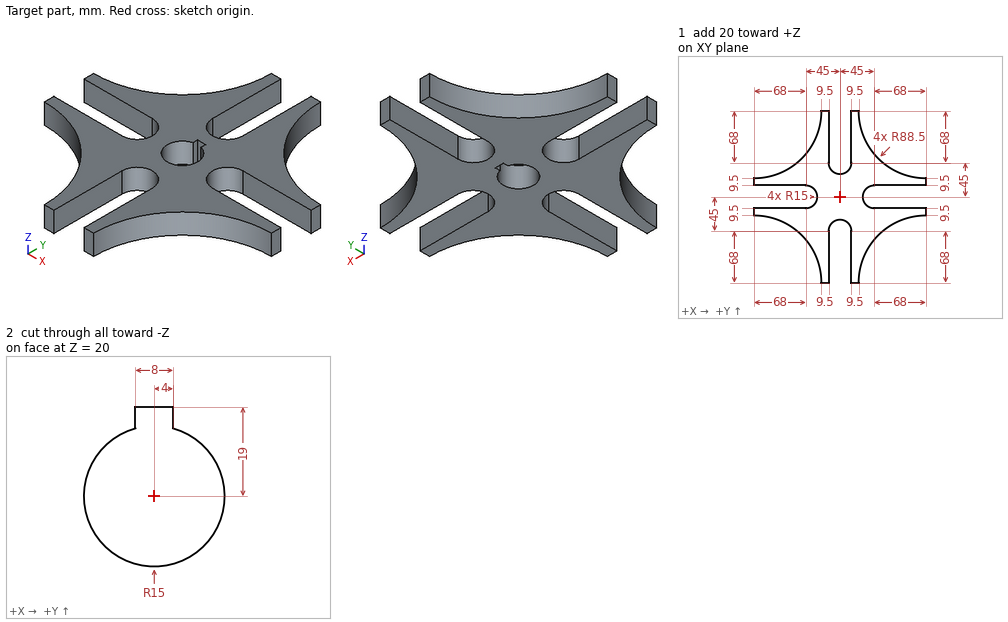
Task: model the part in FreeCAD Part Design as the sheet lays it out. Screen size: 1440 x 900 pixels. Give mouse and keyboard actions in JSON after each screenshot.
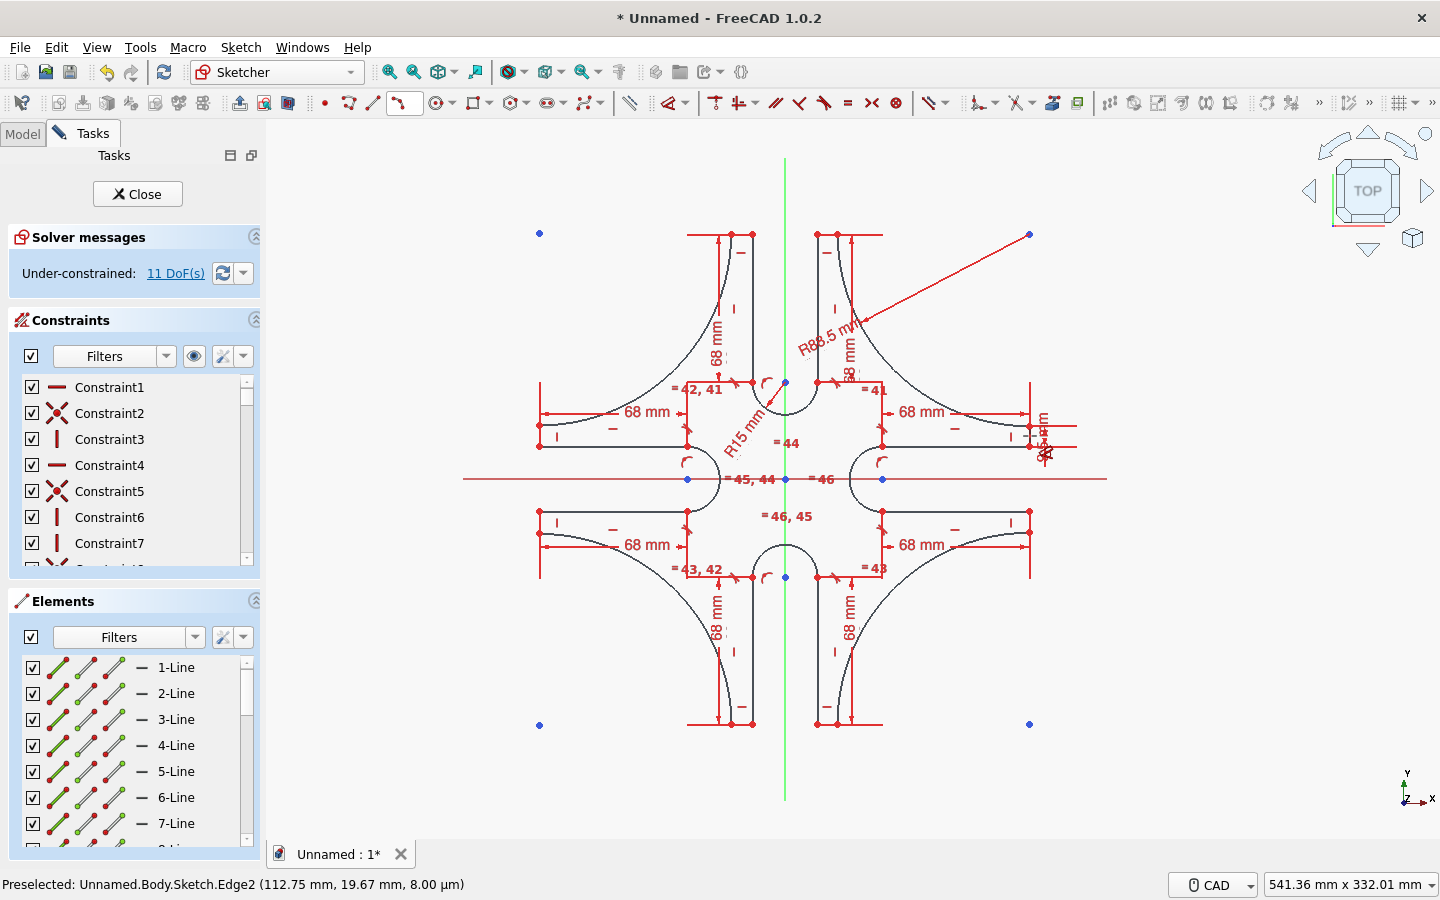
{"action": "scroll", "coordinate": [832, 235], "scroll_direction": "up", "scroll_amount": 5}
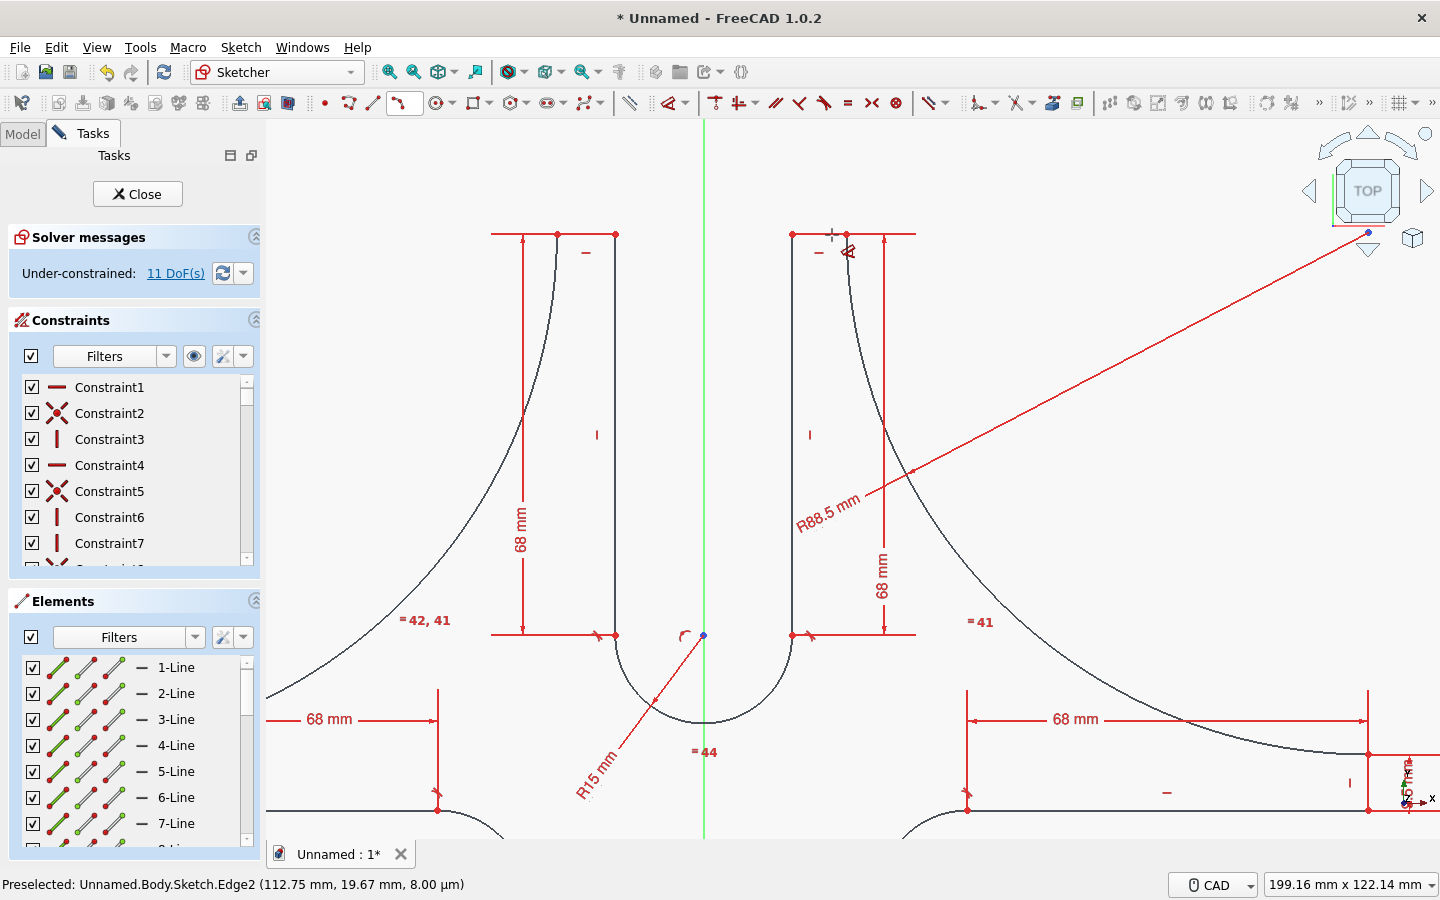
{"action": "left_click", "coordinate": [830, 234]}
{"action": "left_click", "coordinate": [819, 200]}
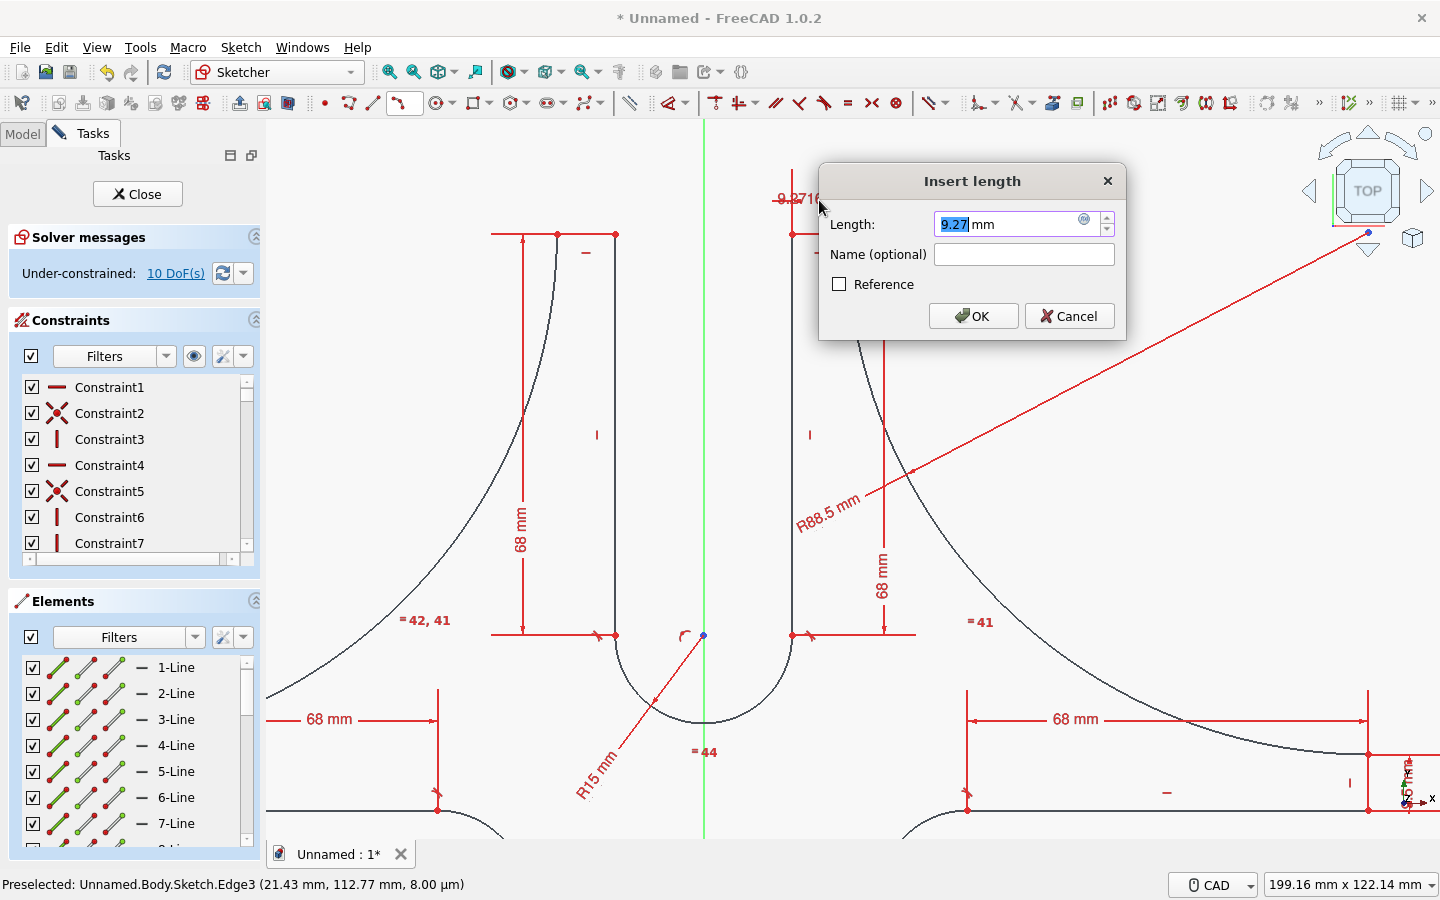
{"action": "type", "text": "9.5"}
{"action": "key", "text": "Return"}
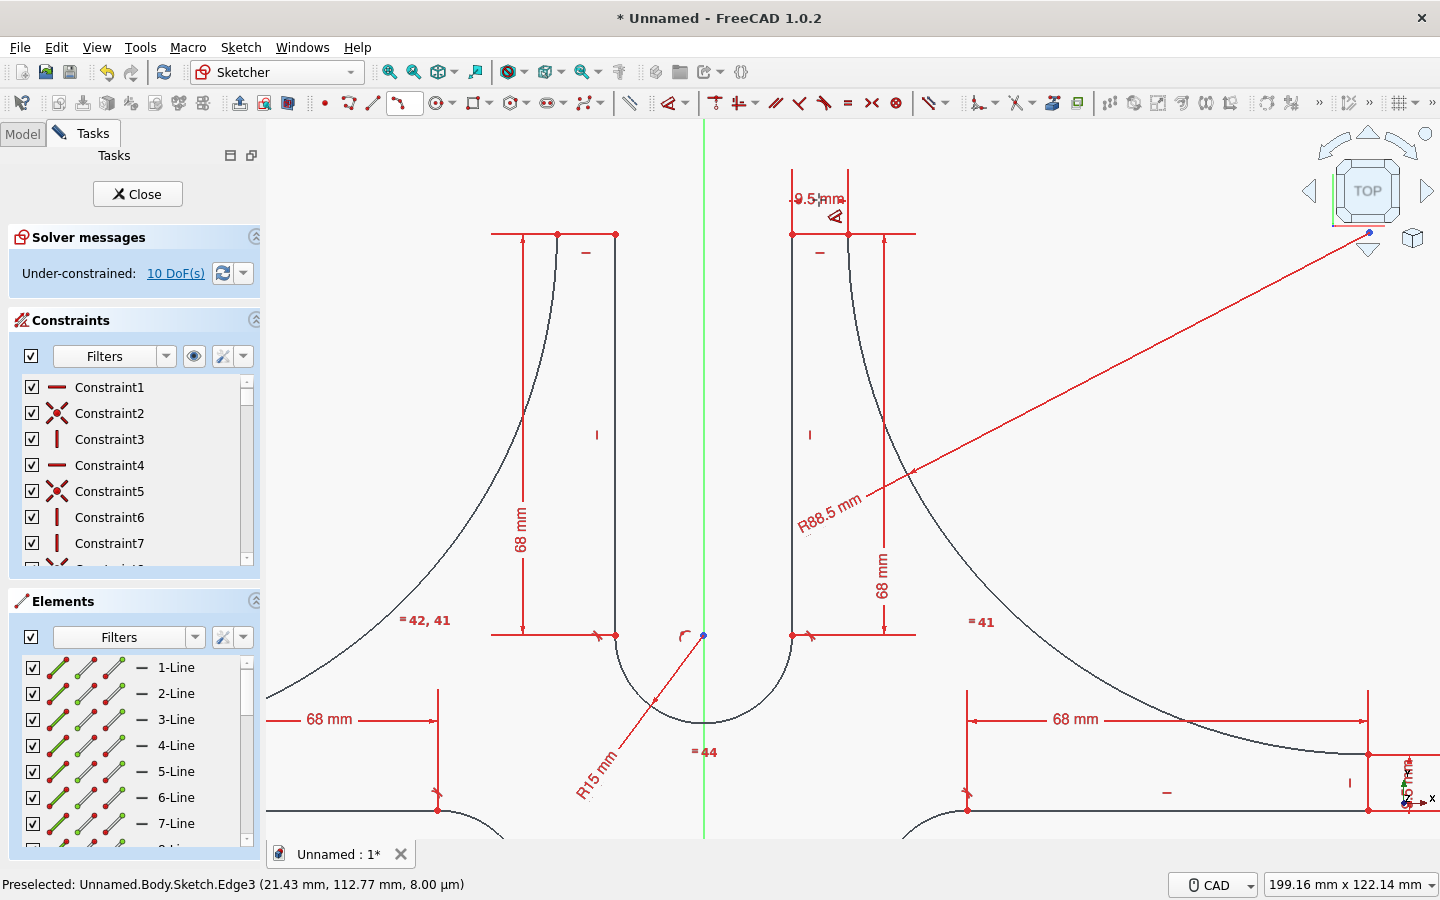
{"action": "left_click", "coordinate": [598, 234]}
{"action": "left_click", "coordinate": [586, 200]}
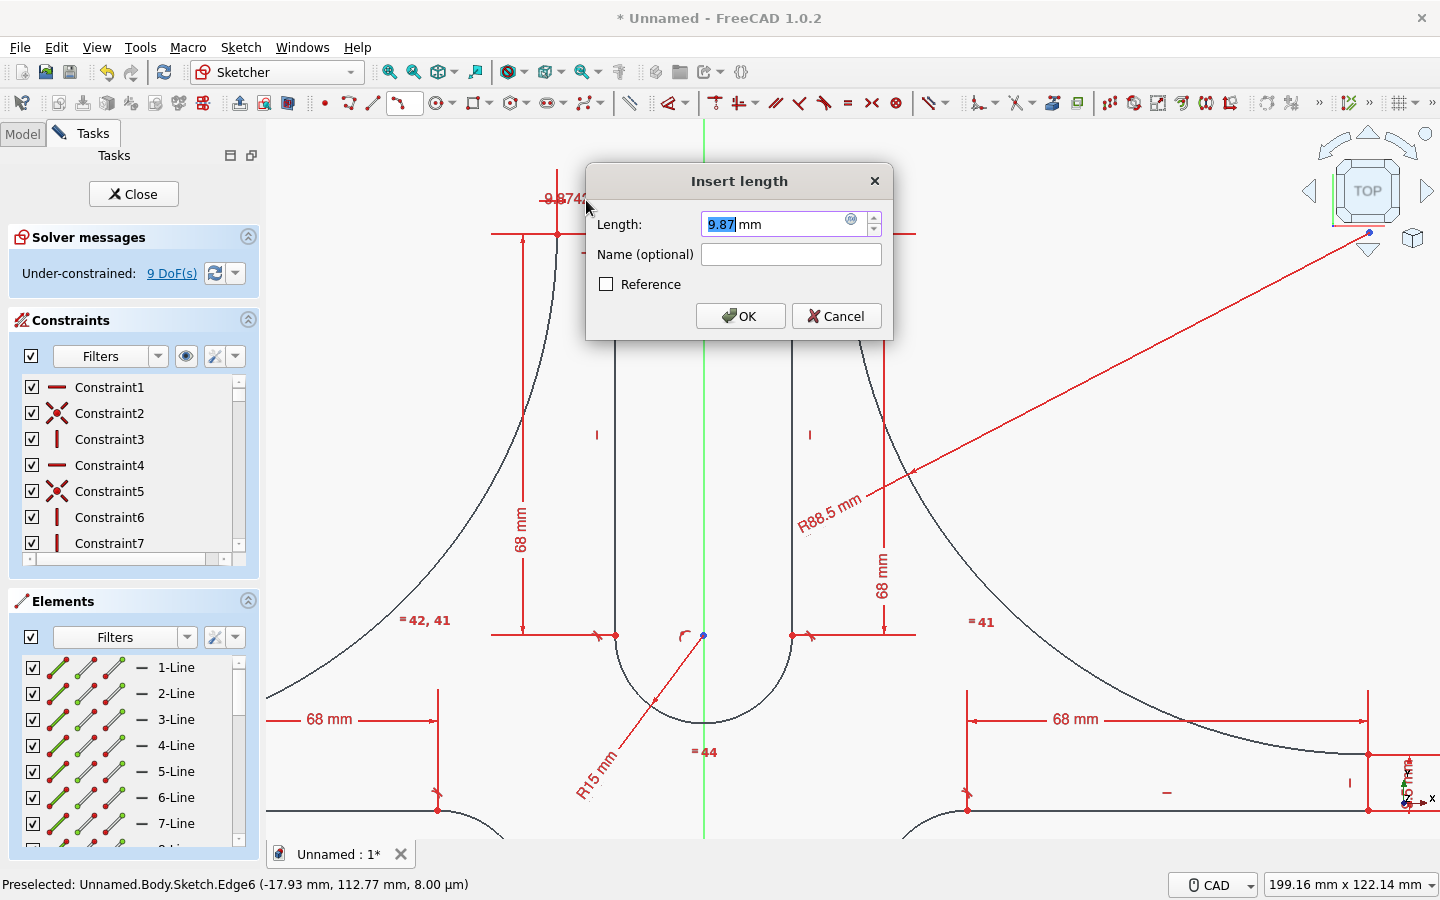
{"action": "type", "text": "9.5"}
{"action": "key", "text": "Return"}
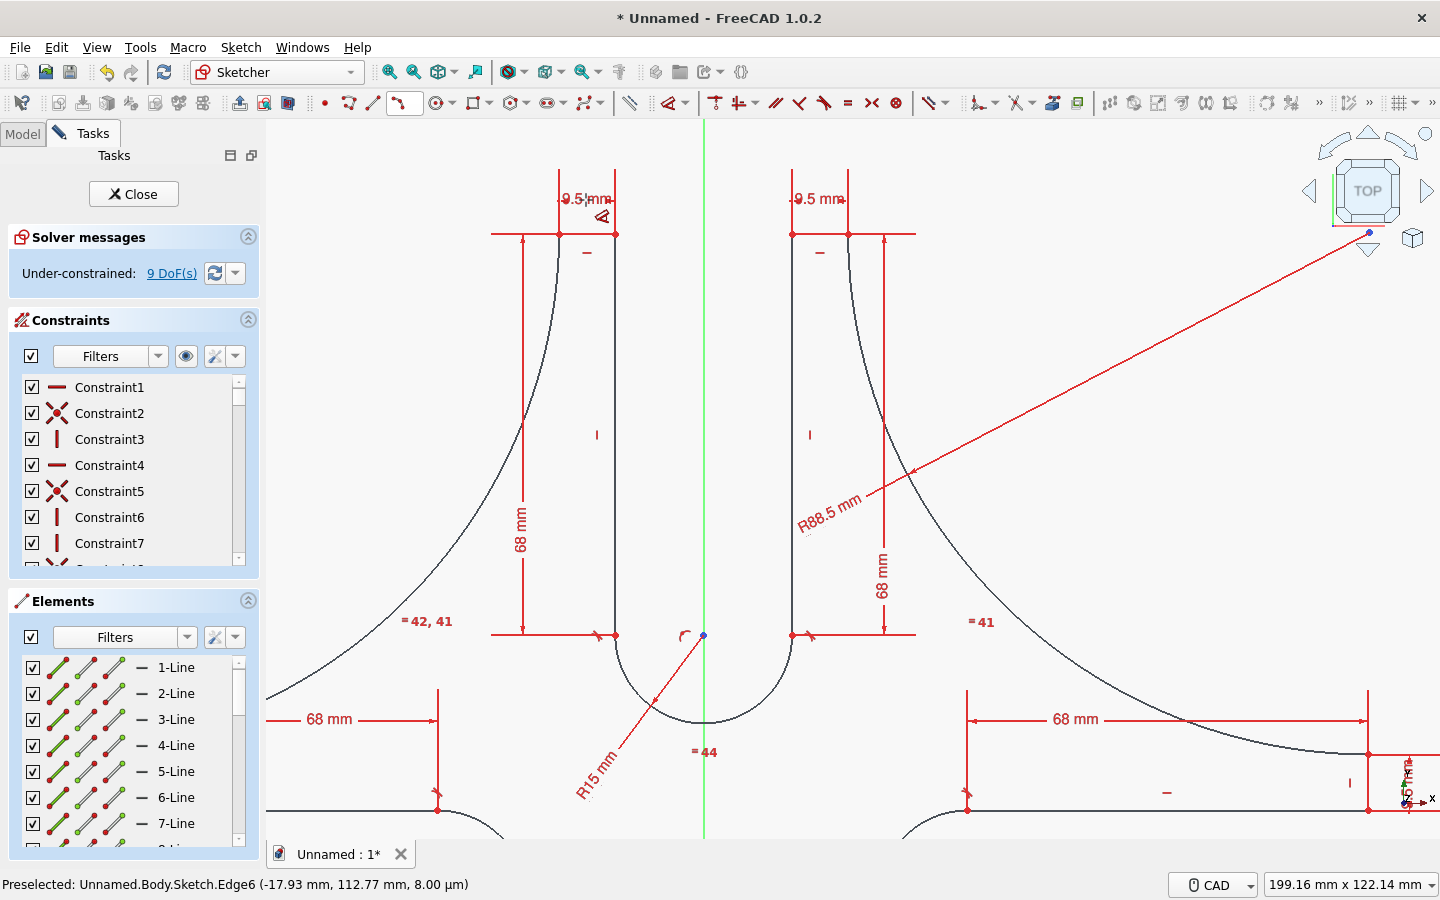
{"action": "scroll", "coordinate": [832, 235], "scroll_direction": "down", "scroll_amount": 5}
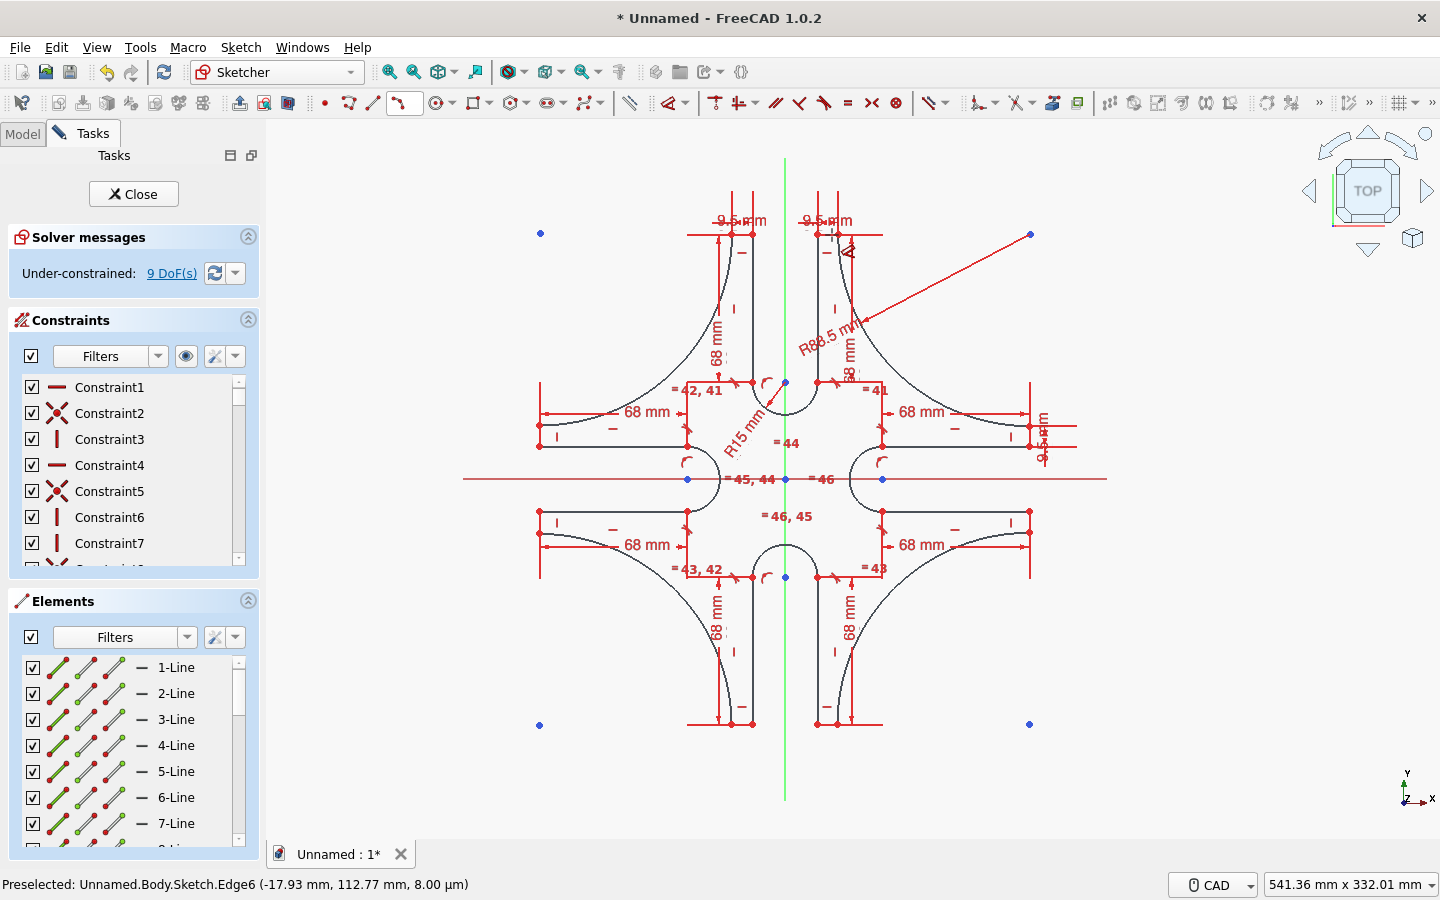
{"action": "scroll", "coordinate": [540, 432], "scroll_direction": "up", "scroll_amount": 4}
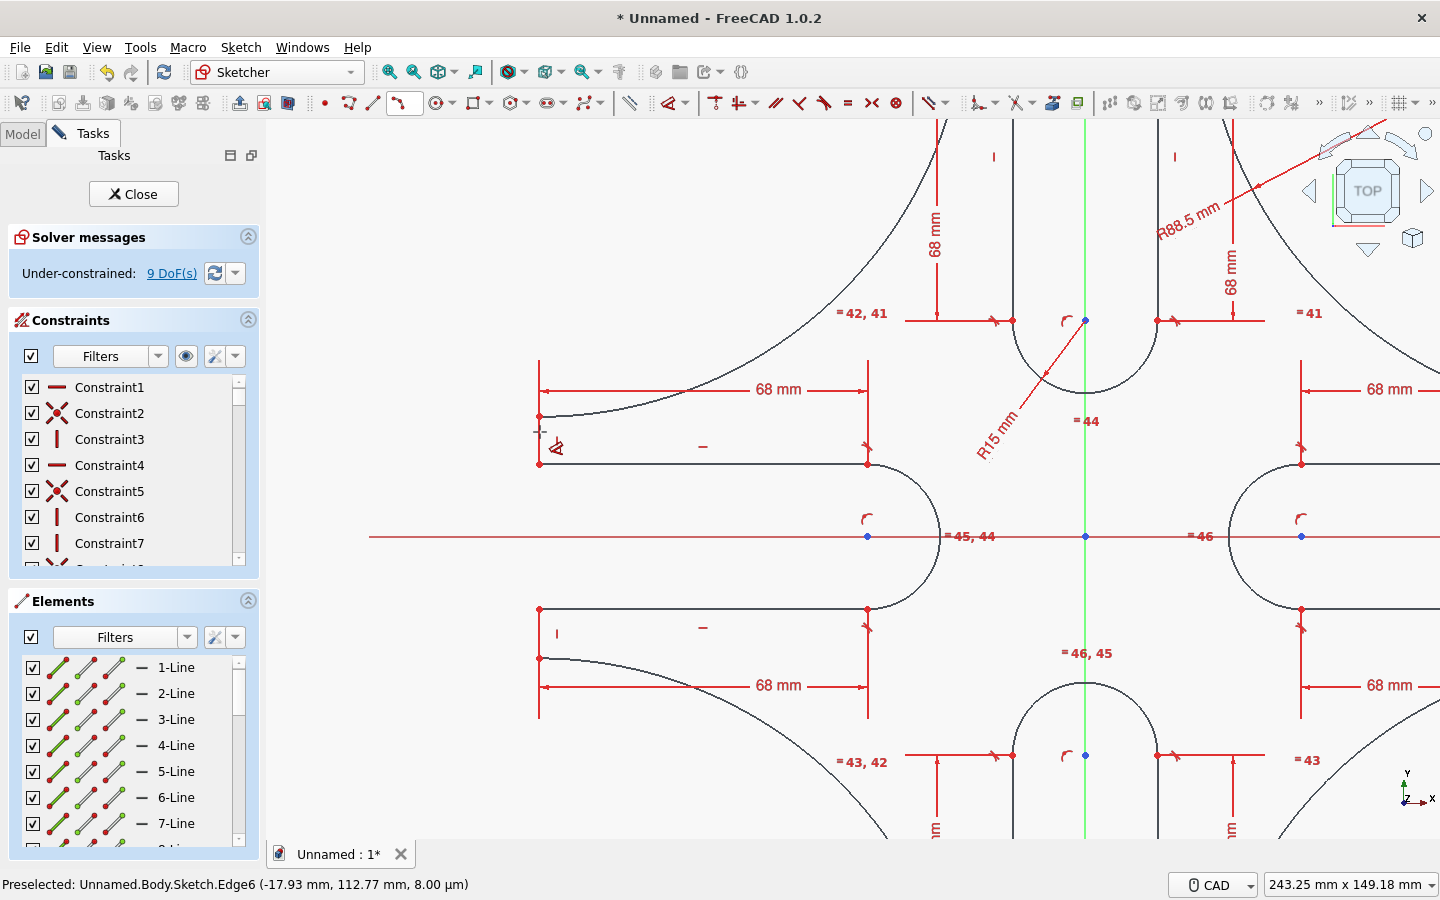
{"action": "left_click", "coordinate": [539, 431]}
{"action": "left_click", "coordinate": [505, 441]}